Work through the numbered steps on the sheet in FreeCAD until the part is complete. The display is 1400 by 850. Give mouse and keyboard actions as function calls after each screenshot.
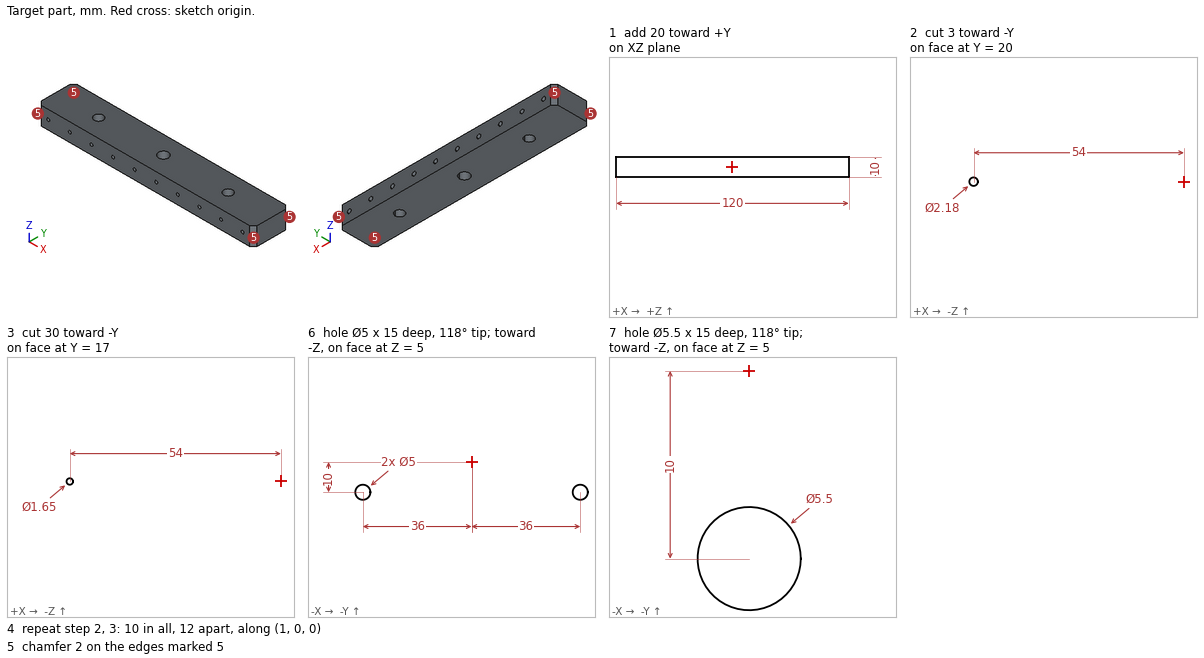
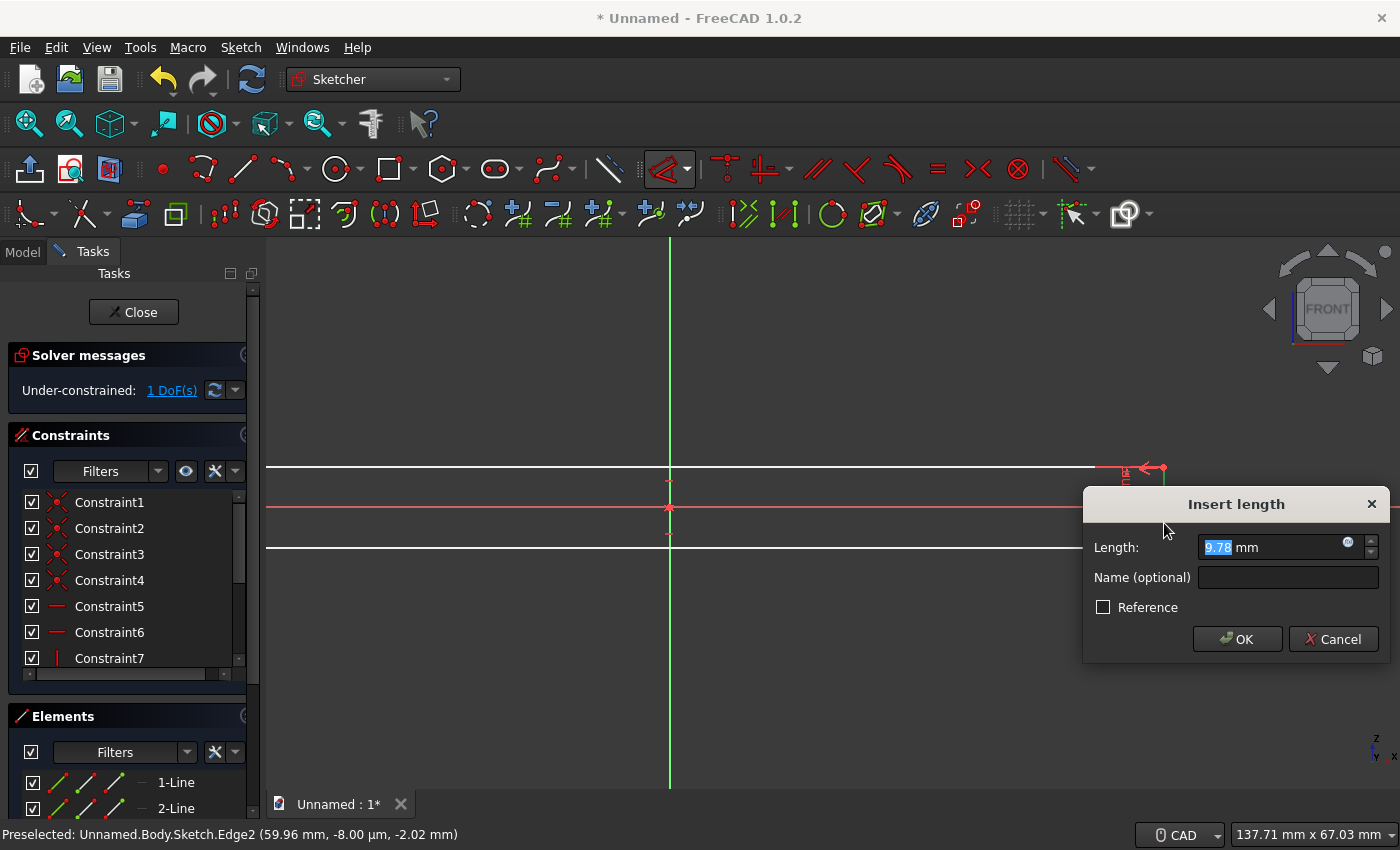
text(10)
key(Return)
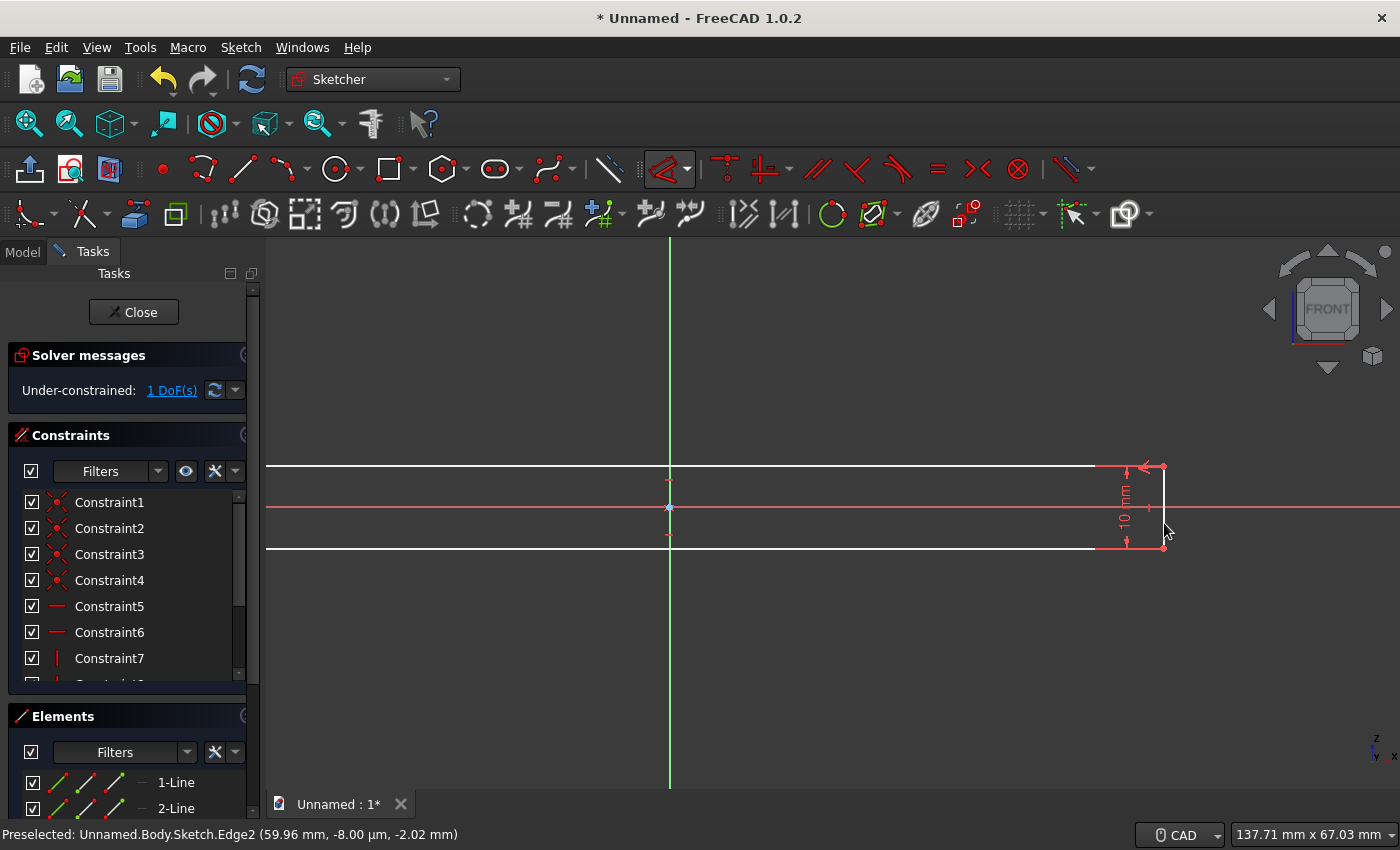
click(472, 549)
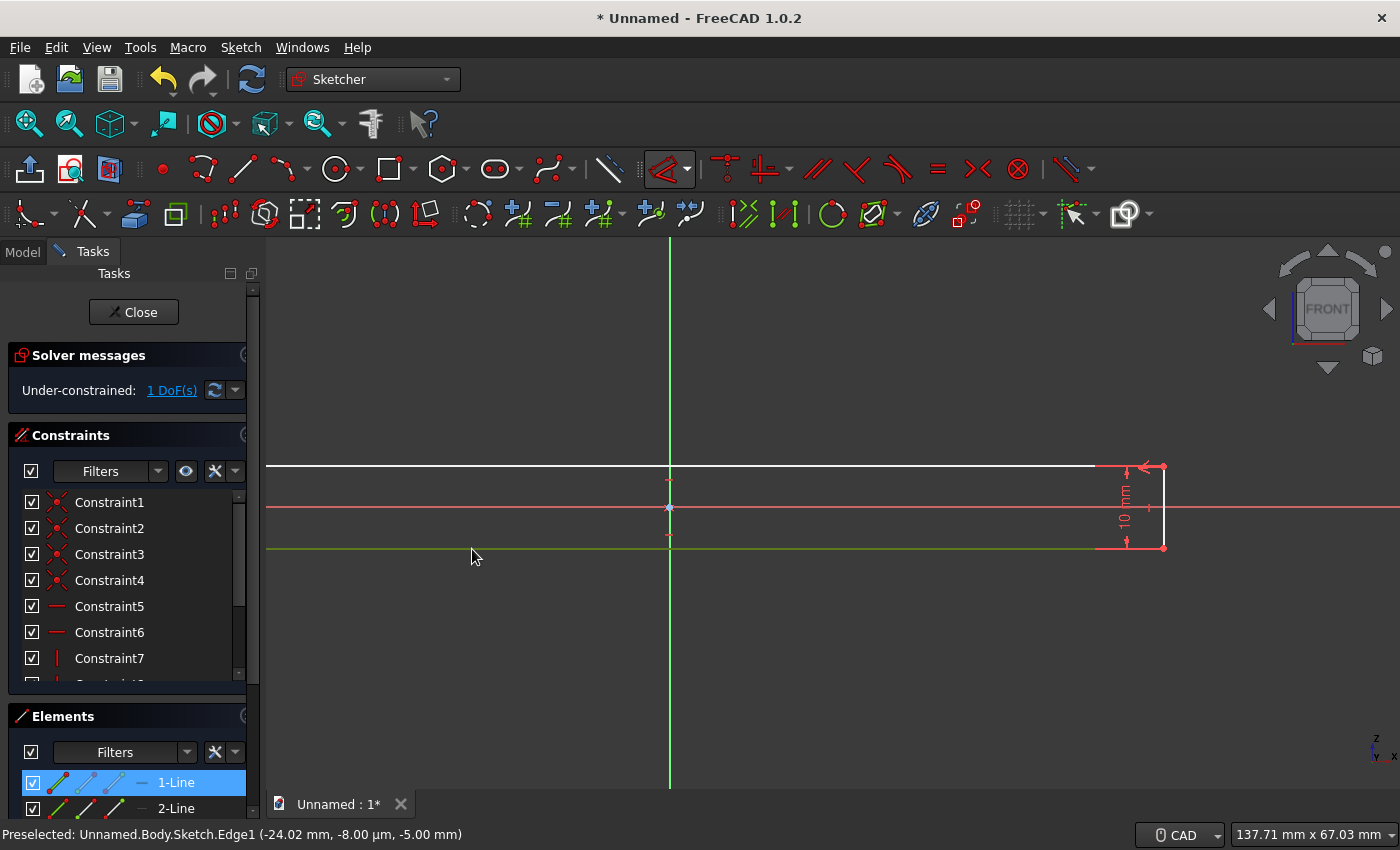
key(l)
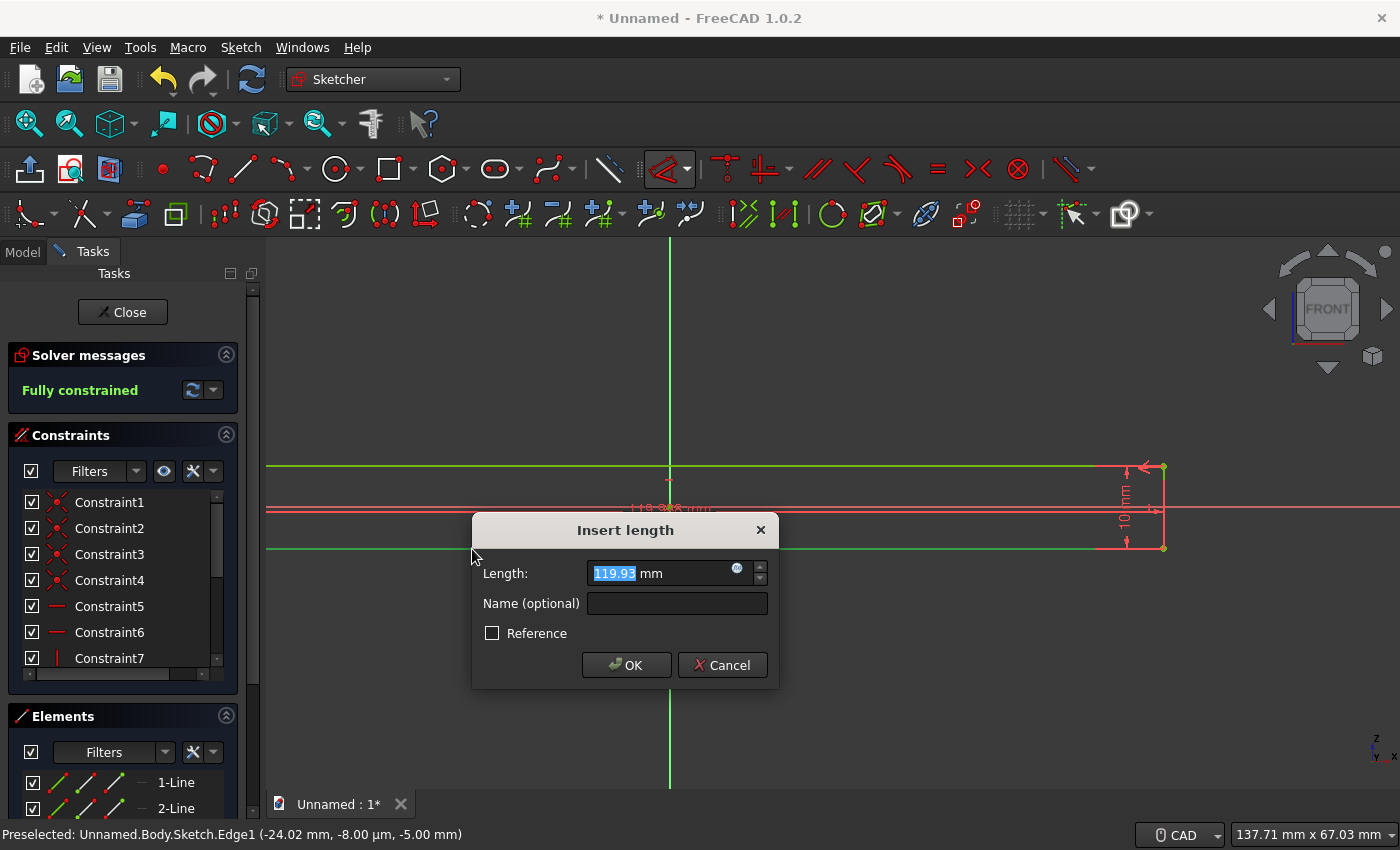
text(120)
key(Return)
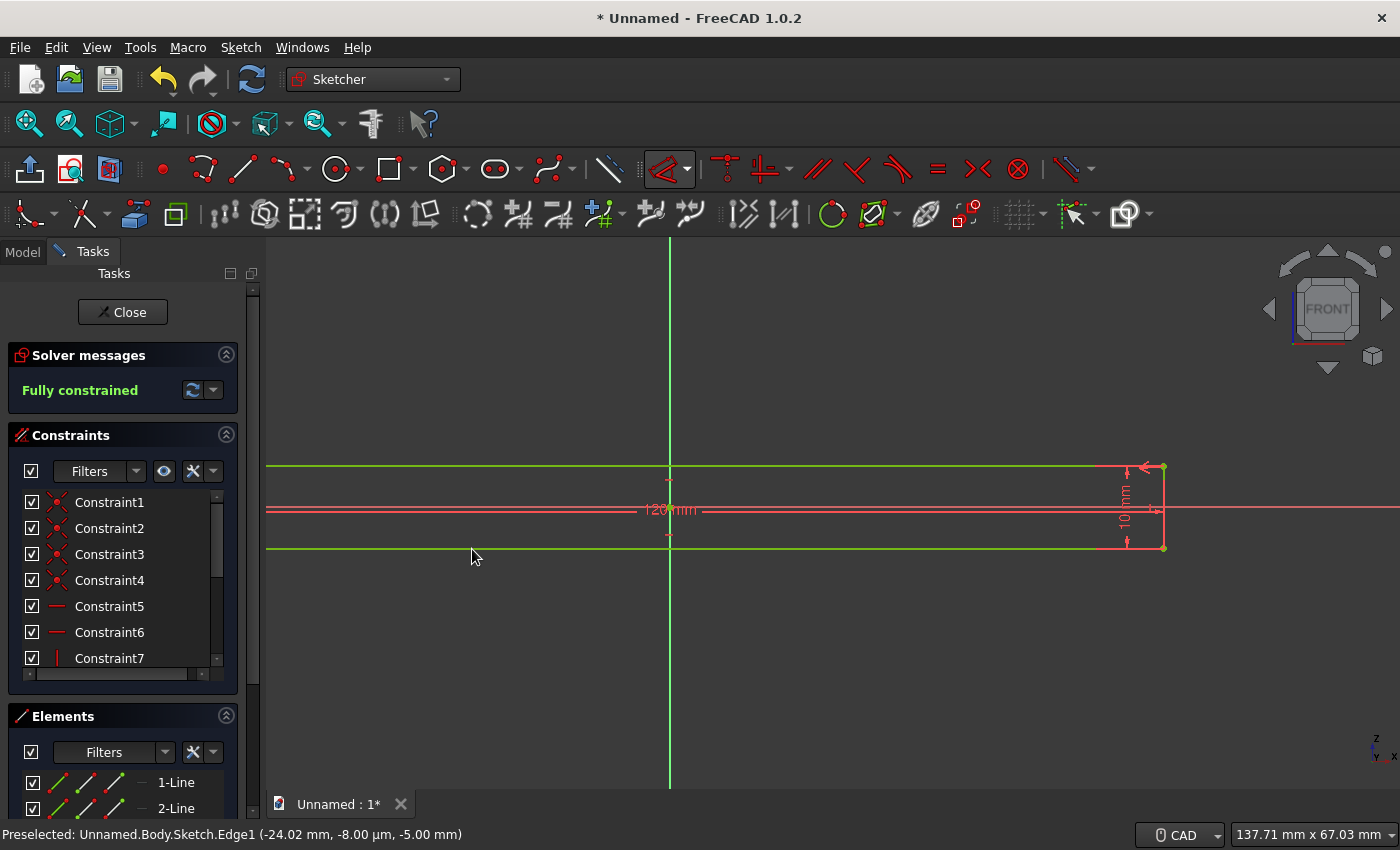
click(123, 312)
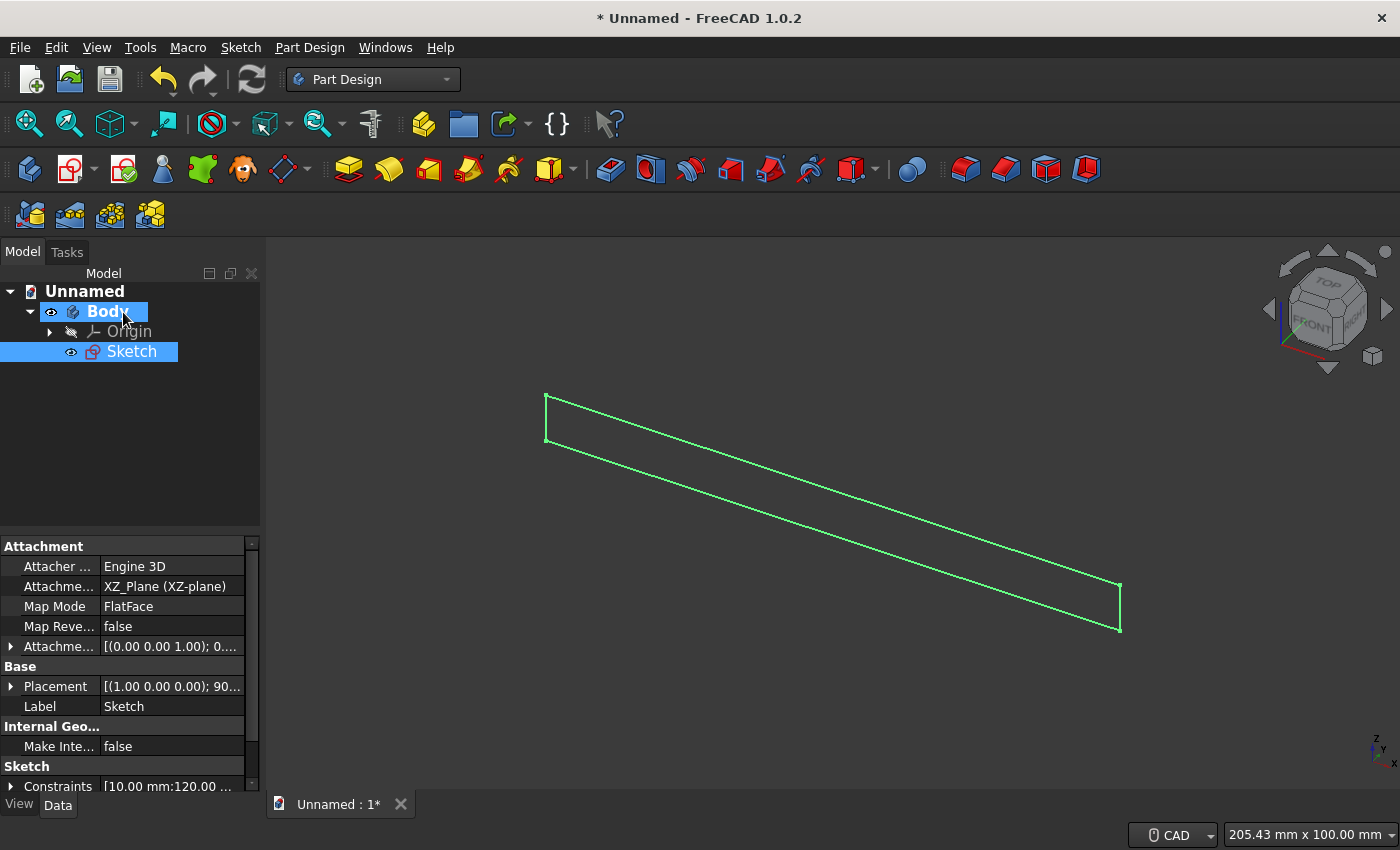
click(350, 170)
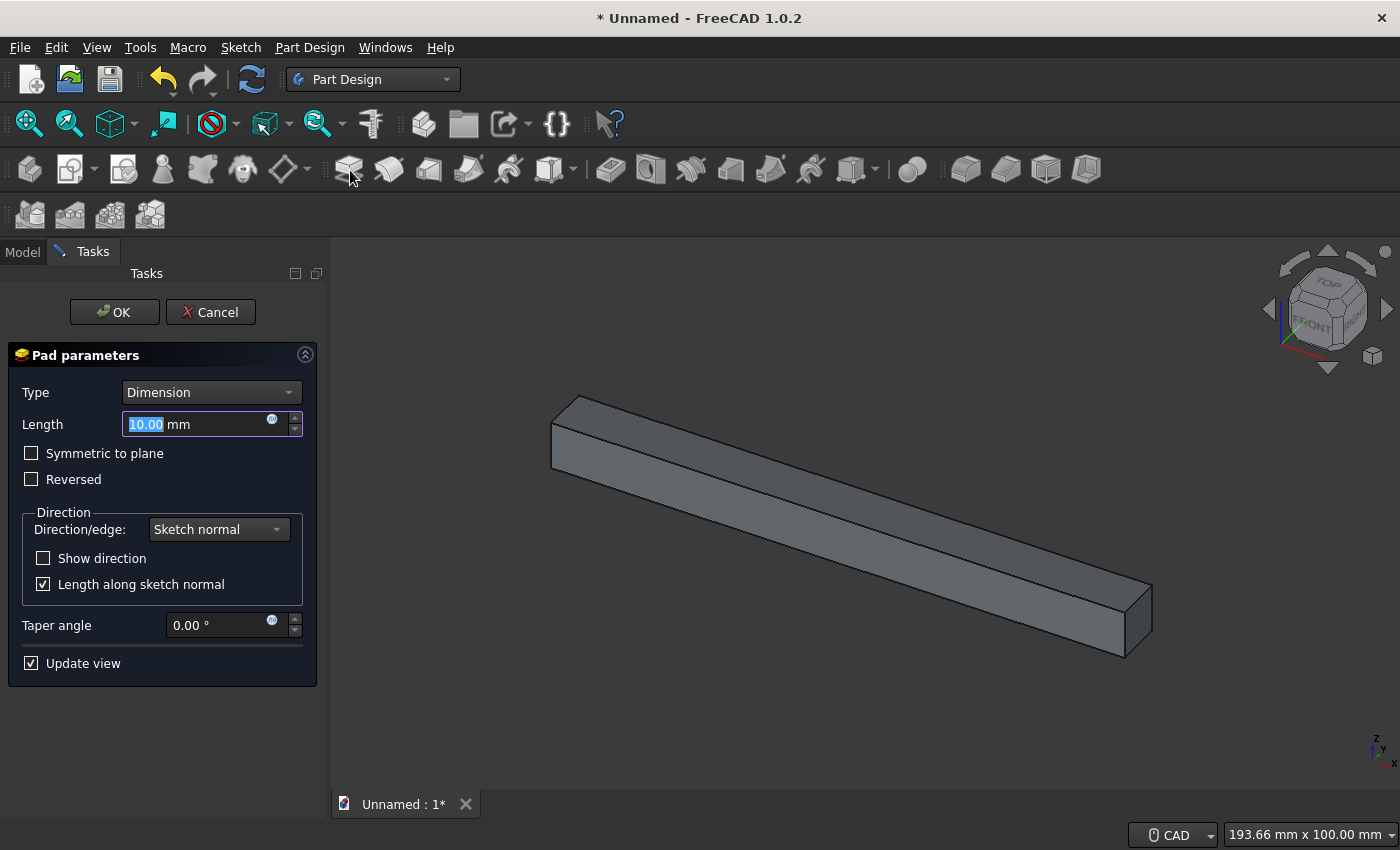
text(20)
key(Tab)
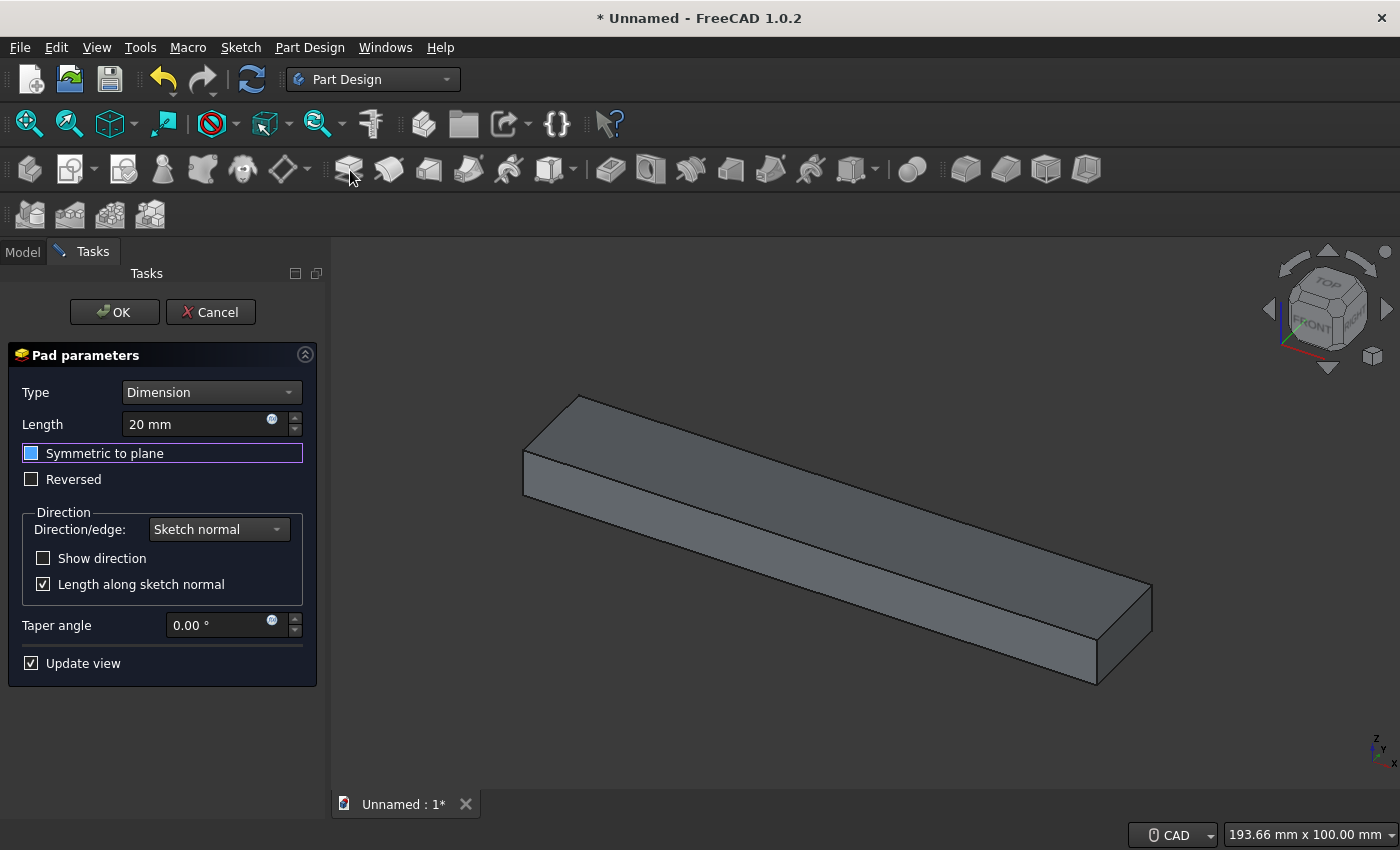
click(30, 479)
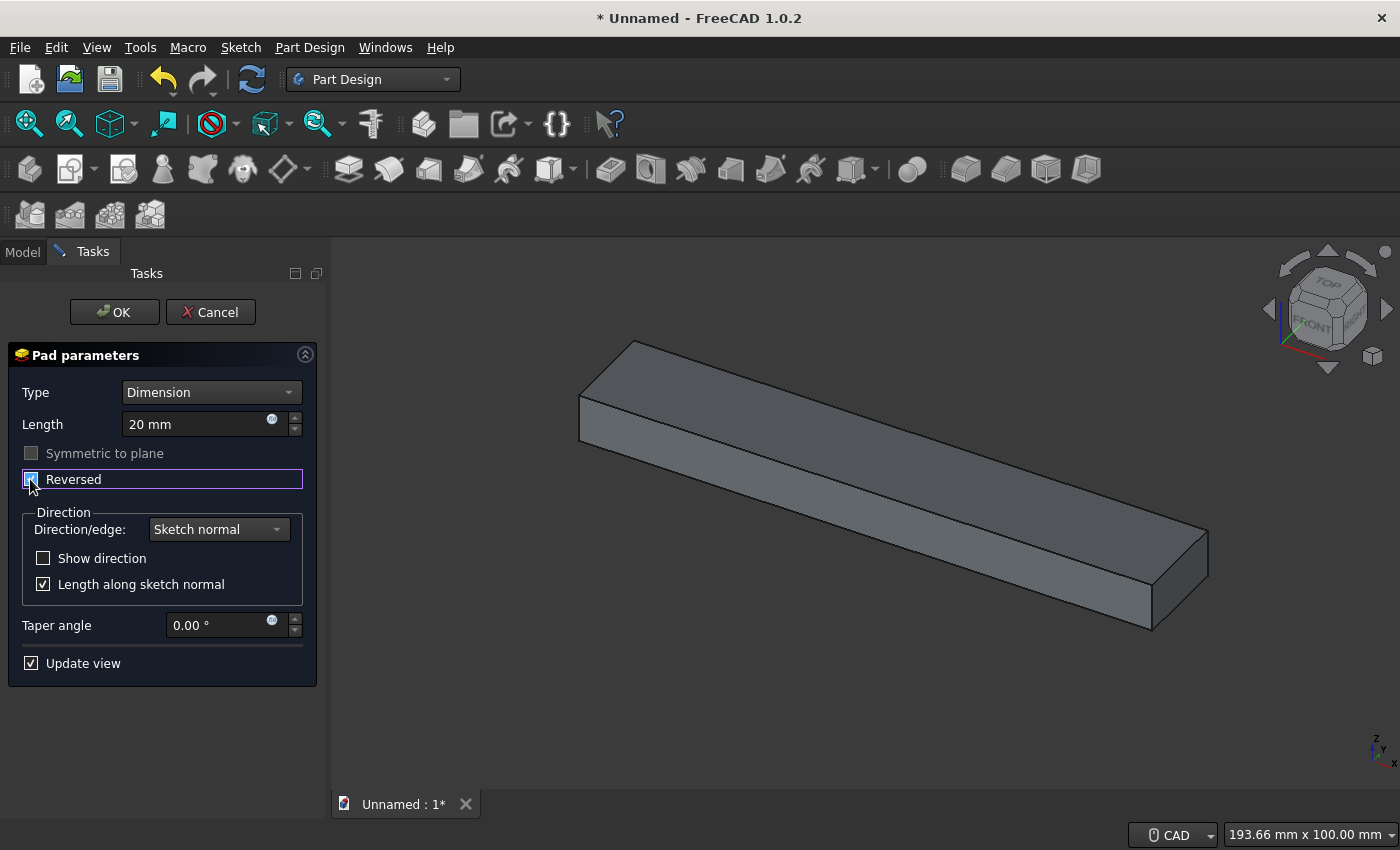
click(115, 312)